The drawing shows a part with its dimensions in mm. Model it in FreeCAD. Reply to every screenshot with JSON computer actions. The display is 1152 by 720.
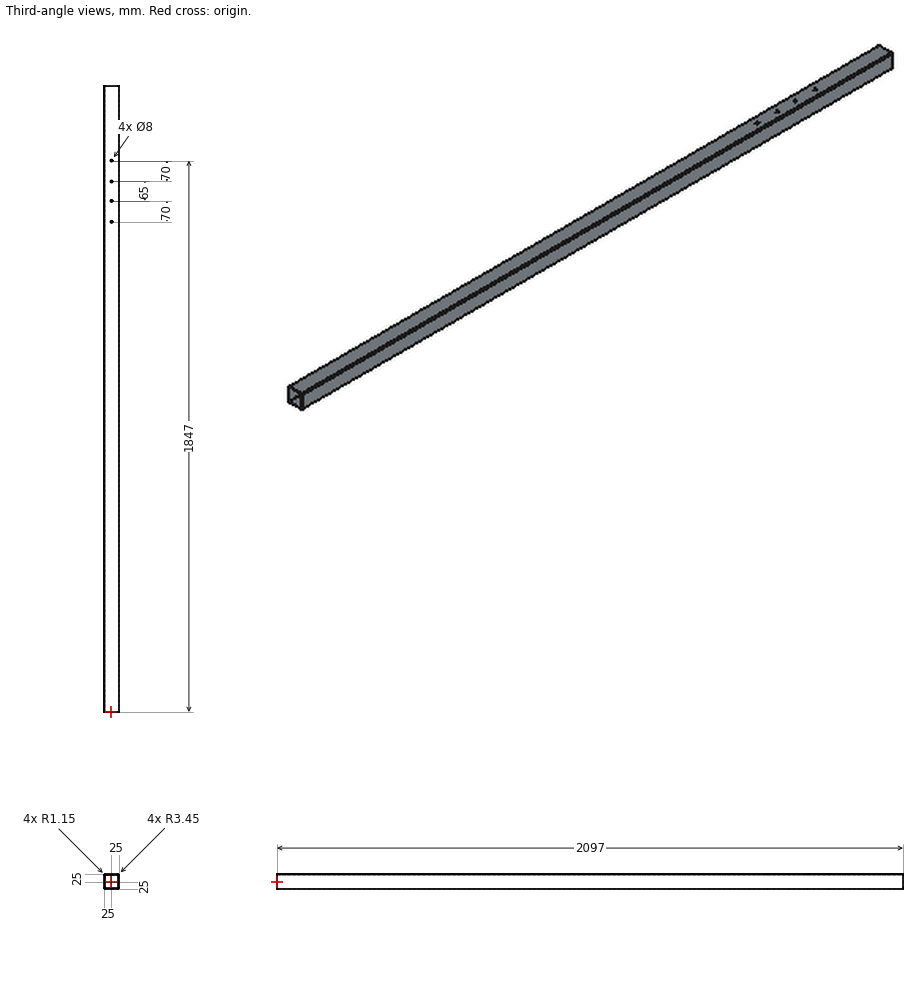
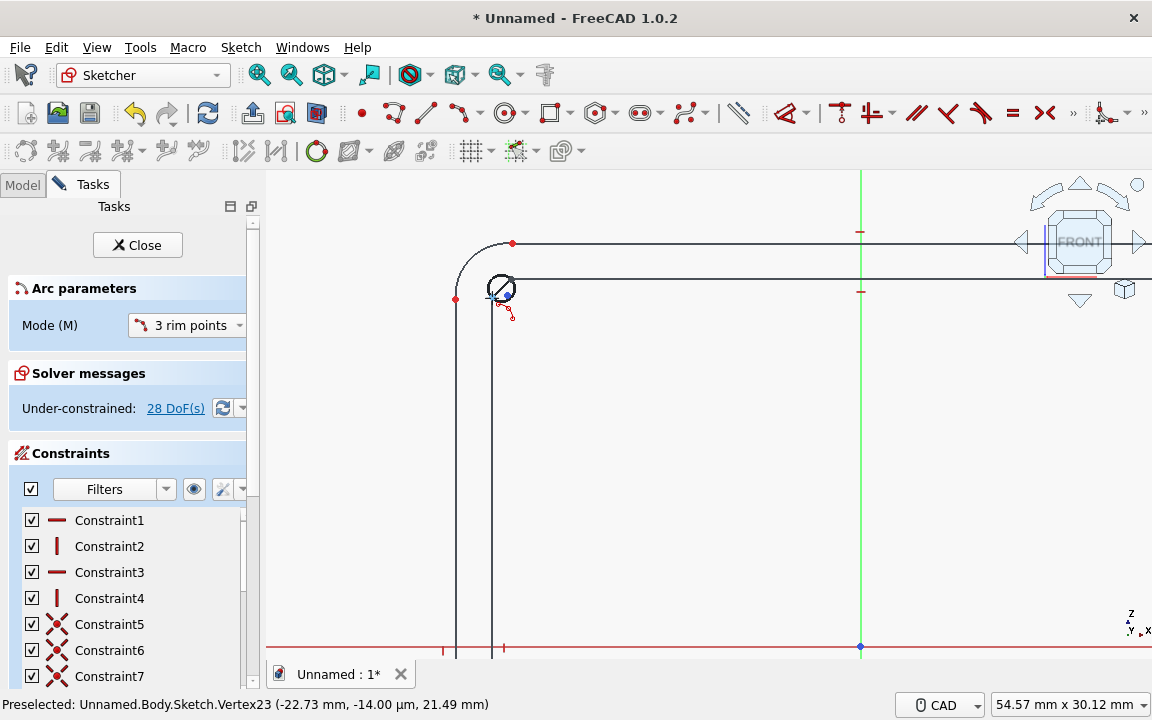
{"action": "scroll", "coordinate": [498, 284], "scroll_direction": "up", "scroll_amount": 6}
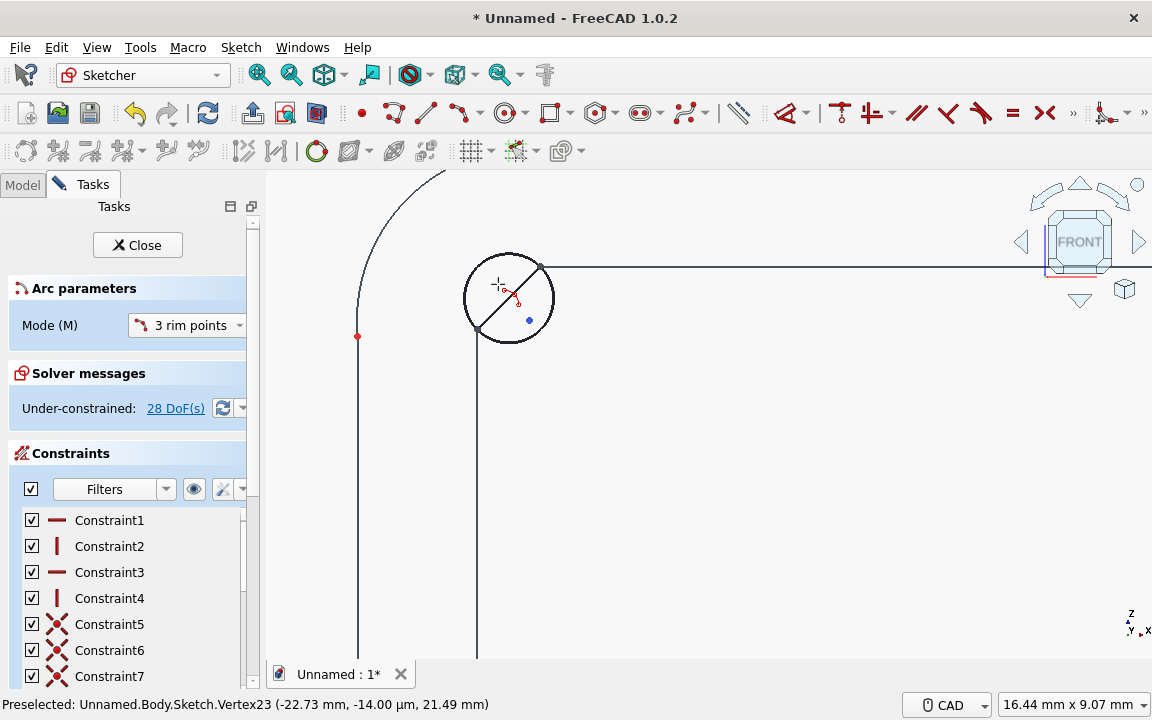
{"action": "left_click", "coordinate": [497, 283]}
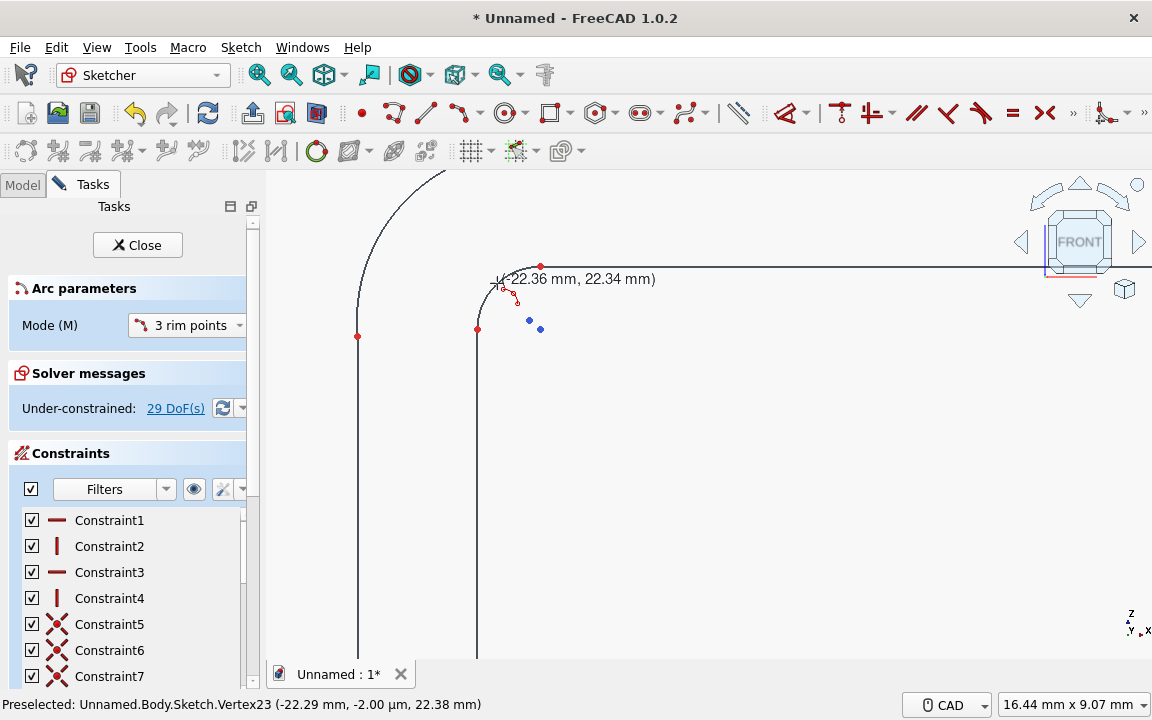
{"action": "scroll", "coordinate": [508, 281], "scroll_direction": "down", "scroll_amount": 11}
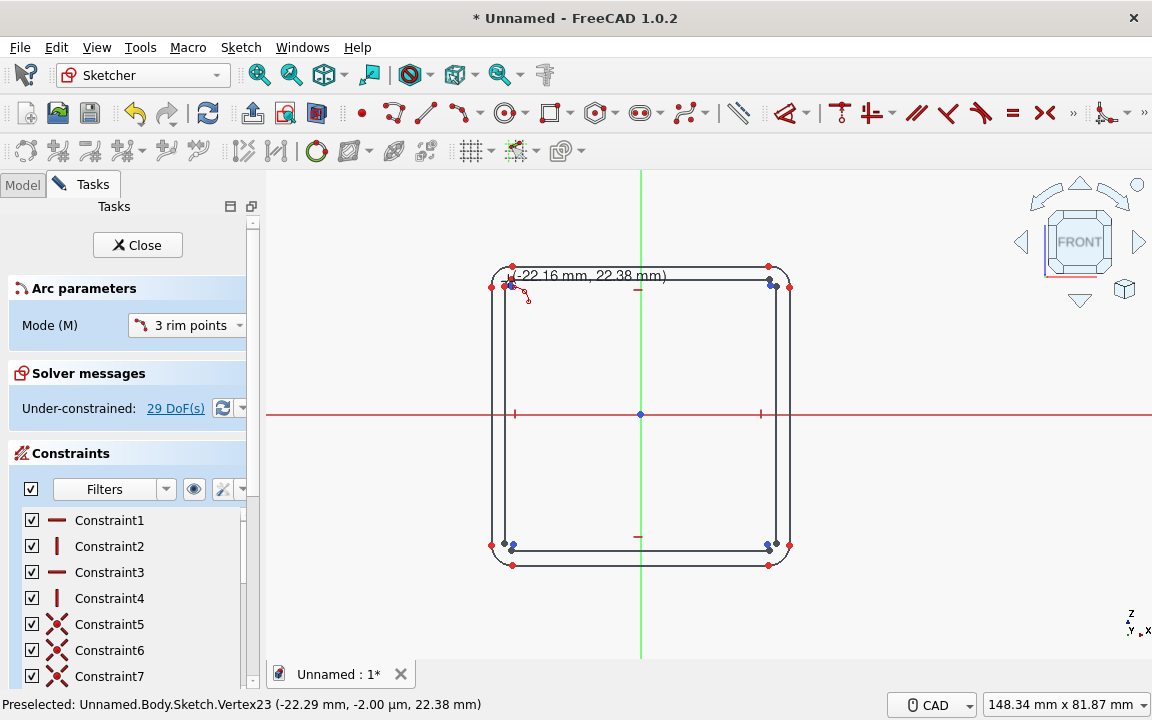
{"action": "scroll", "coordinate": [505, 544], "scroll_direction": "up", "scroll_amount": 5}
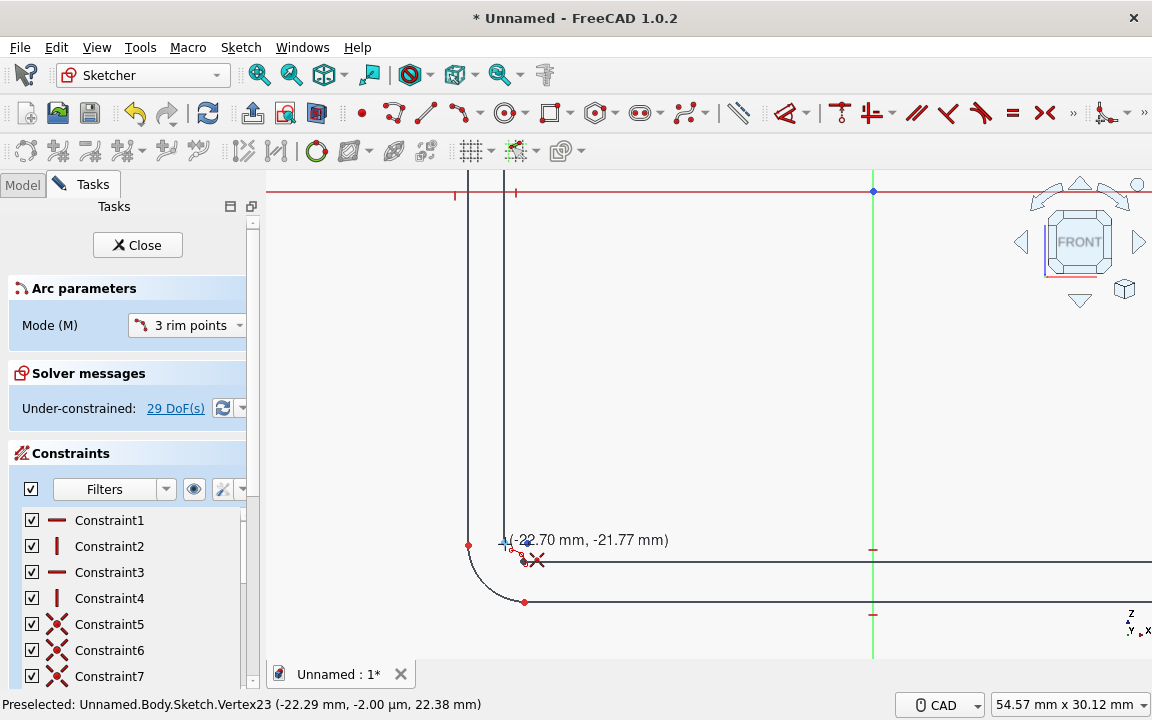
{"action": "left_click", "coordinate": [504, 543]}
{"action": "left_click", "coordinate": [523, 562]}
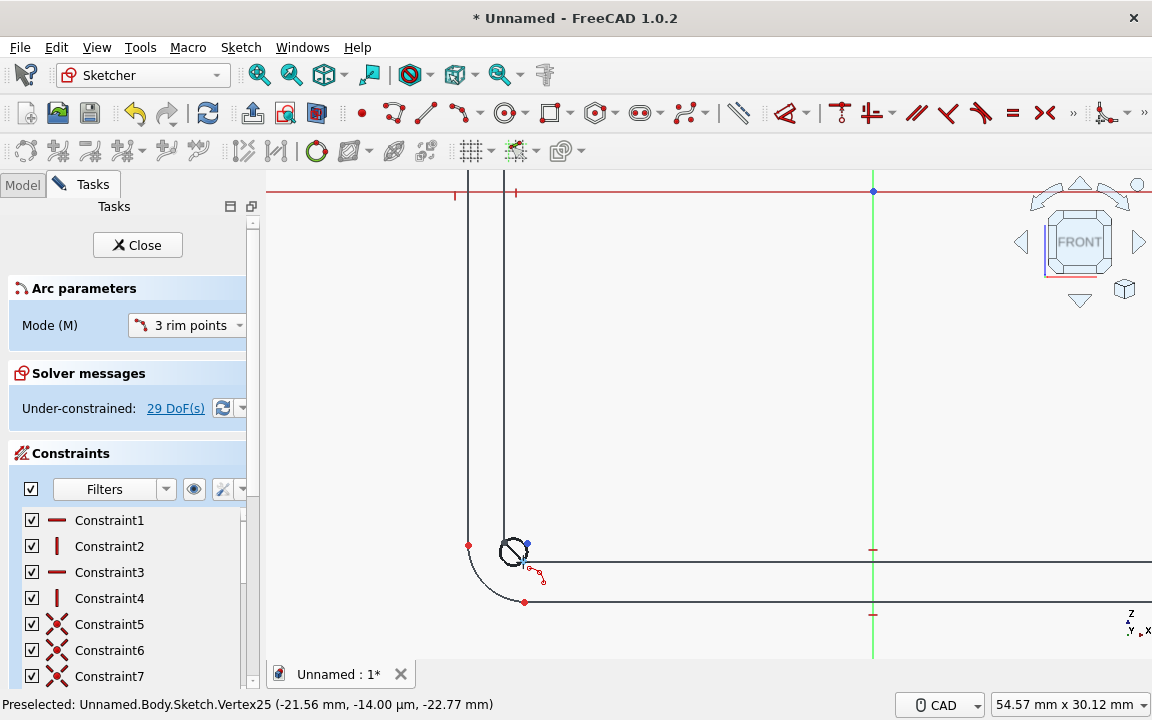
{"action": "scroll", "coordinate": [510, 555], "scroll_direction": "up", "scroll_amount": 6}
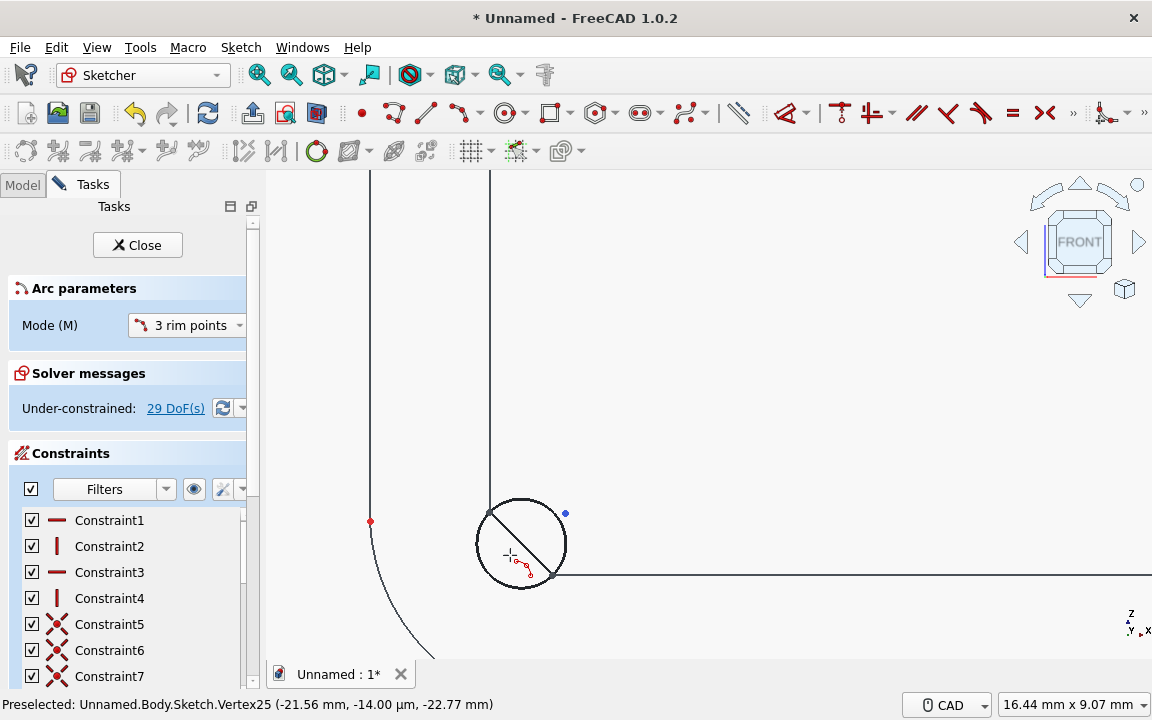
{"action": "left_click", "coordinate": [510, 553]}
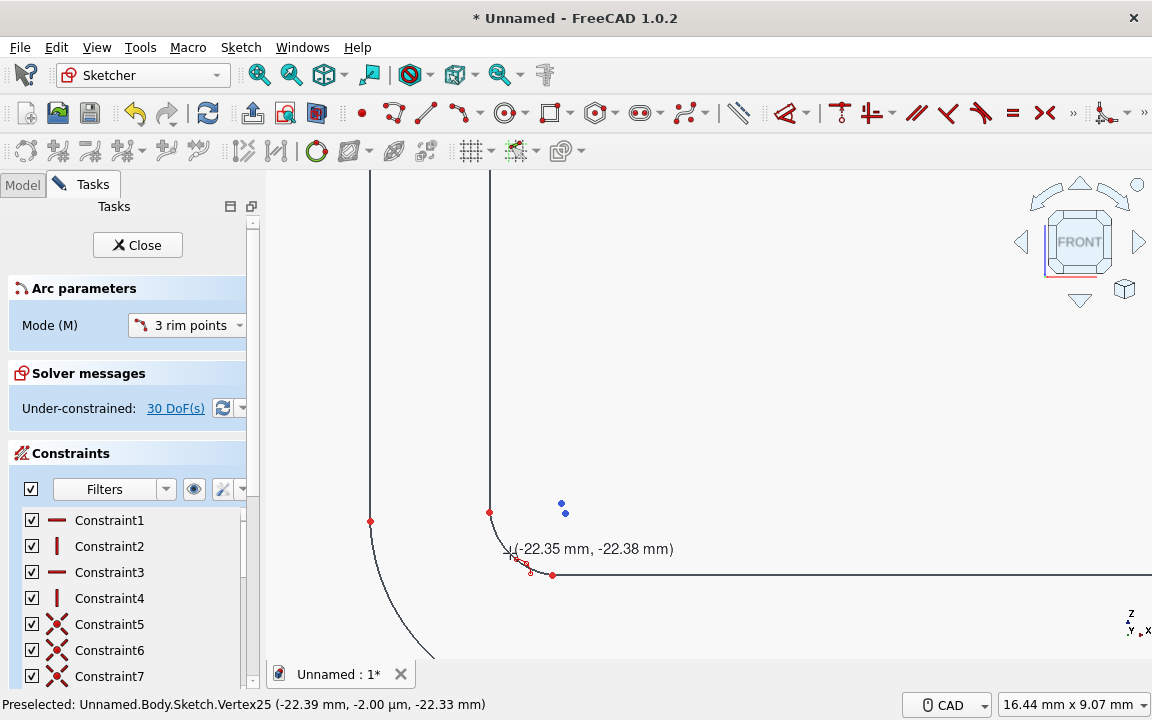
{"action": "scroll", "coordinate": [507, 547], "scroll_direction": "down", "scroll_amount": 11}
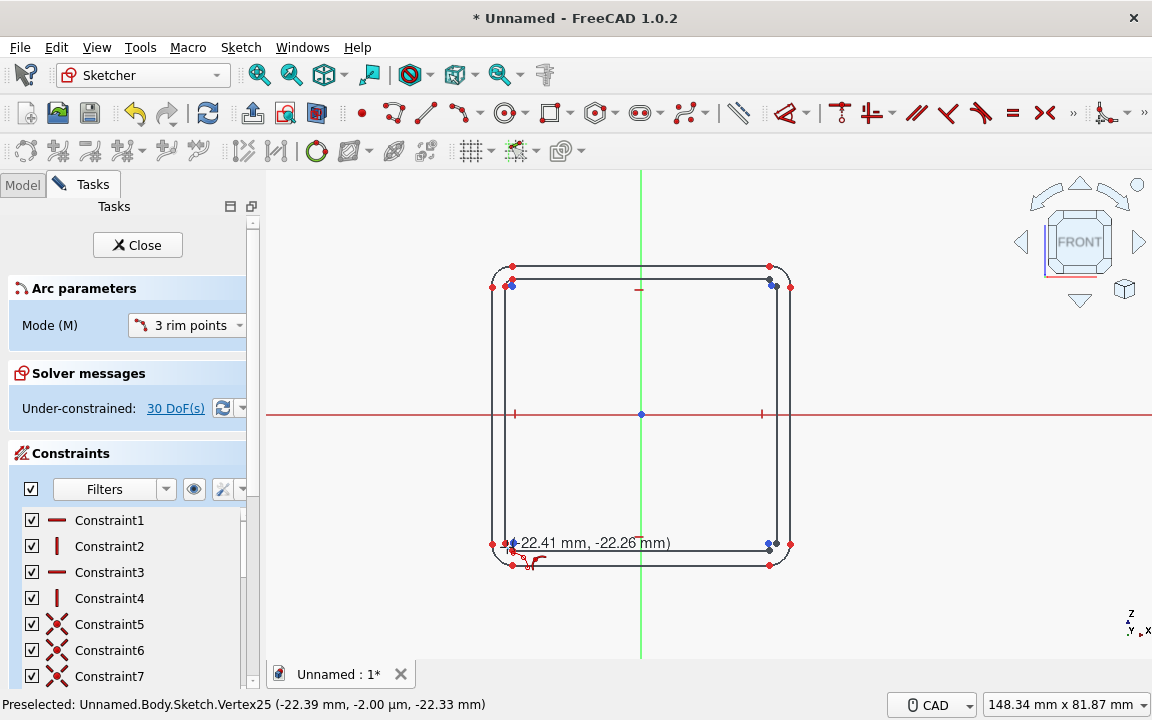
{"action": "scroll", "coordinate": [770, 550], "scroll_direction": "up", "scroll_amount": 5}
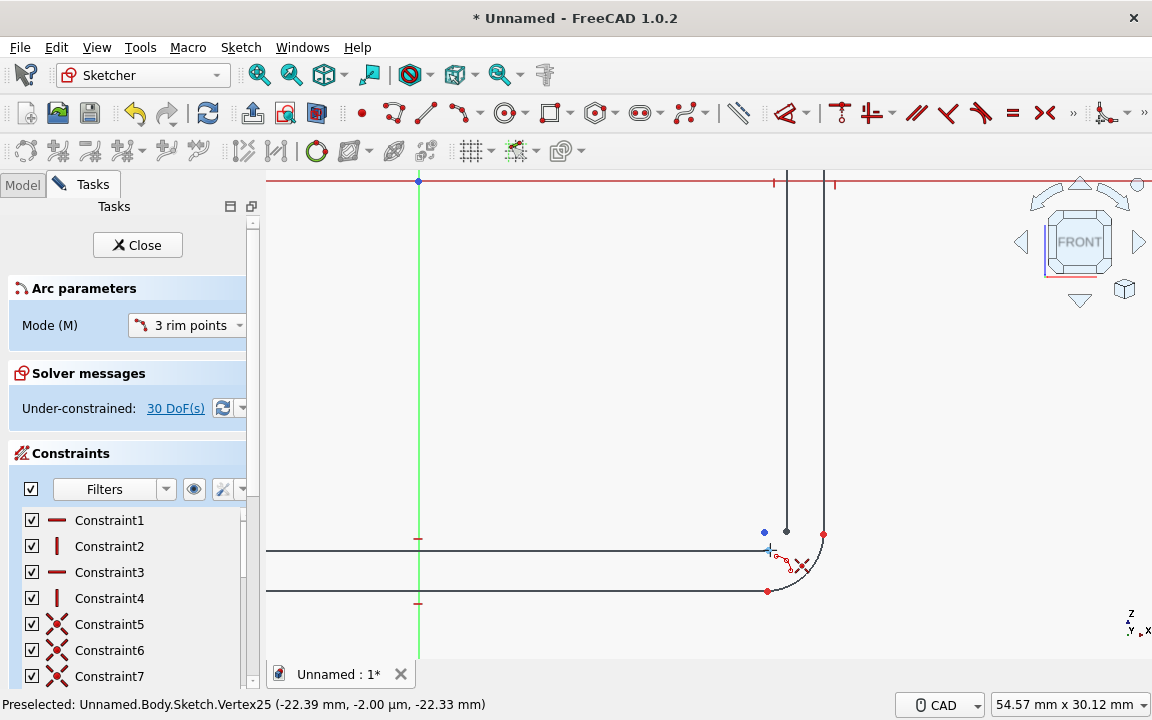
{"action": "left_click", "coordinate": [769, 551]}
{"action": "left_click", "coordinate": [787, 532]}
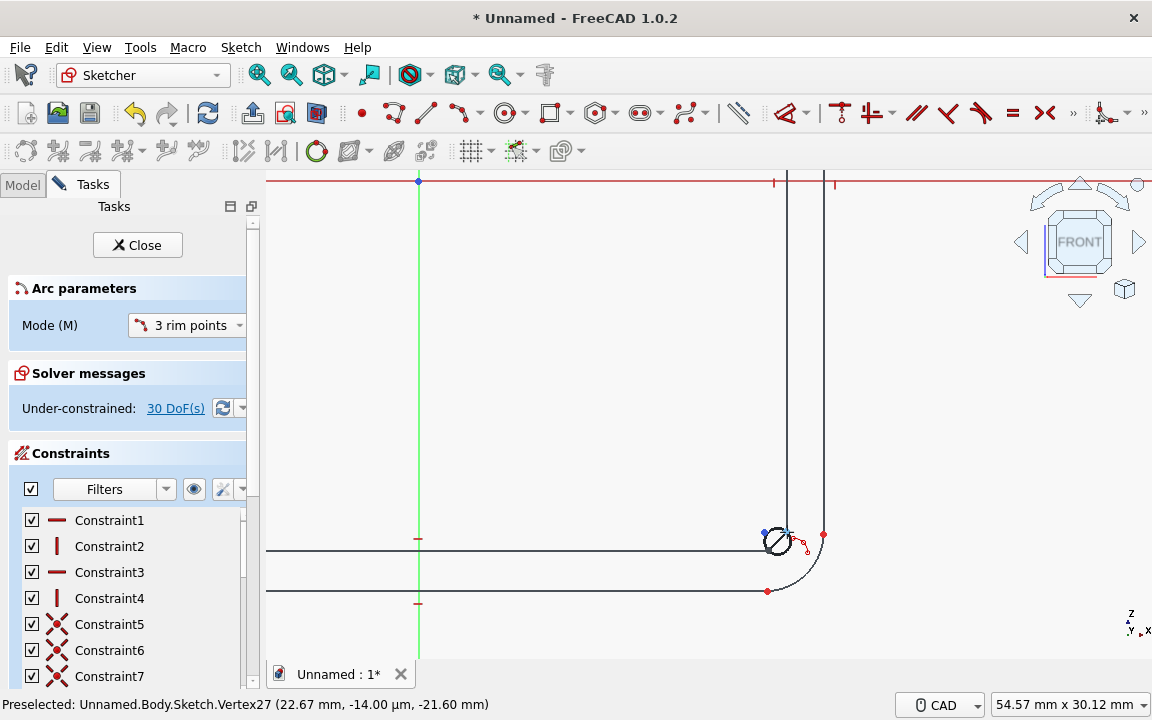
{"action": "scroll", "coordinate": [782, 544], "scroll_direction": "up", "scroll_amount": 6}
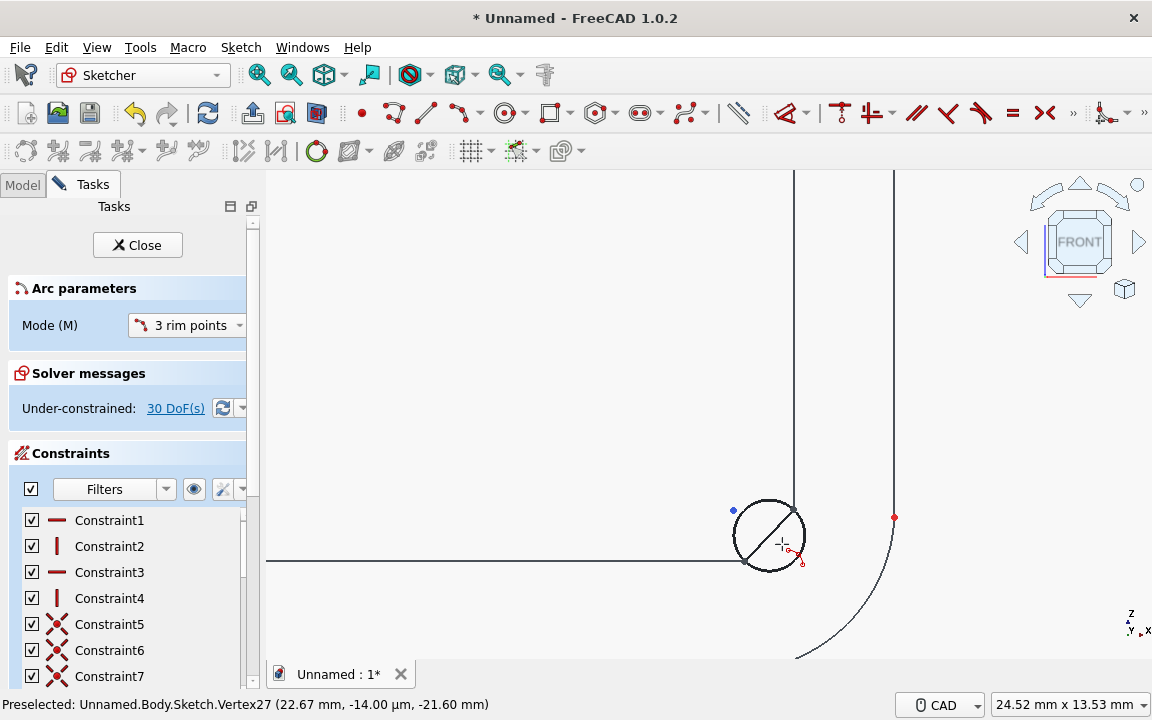
{"action": "left_click", "coordinate": [780, 543]}